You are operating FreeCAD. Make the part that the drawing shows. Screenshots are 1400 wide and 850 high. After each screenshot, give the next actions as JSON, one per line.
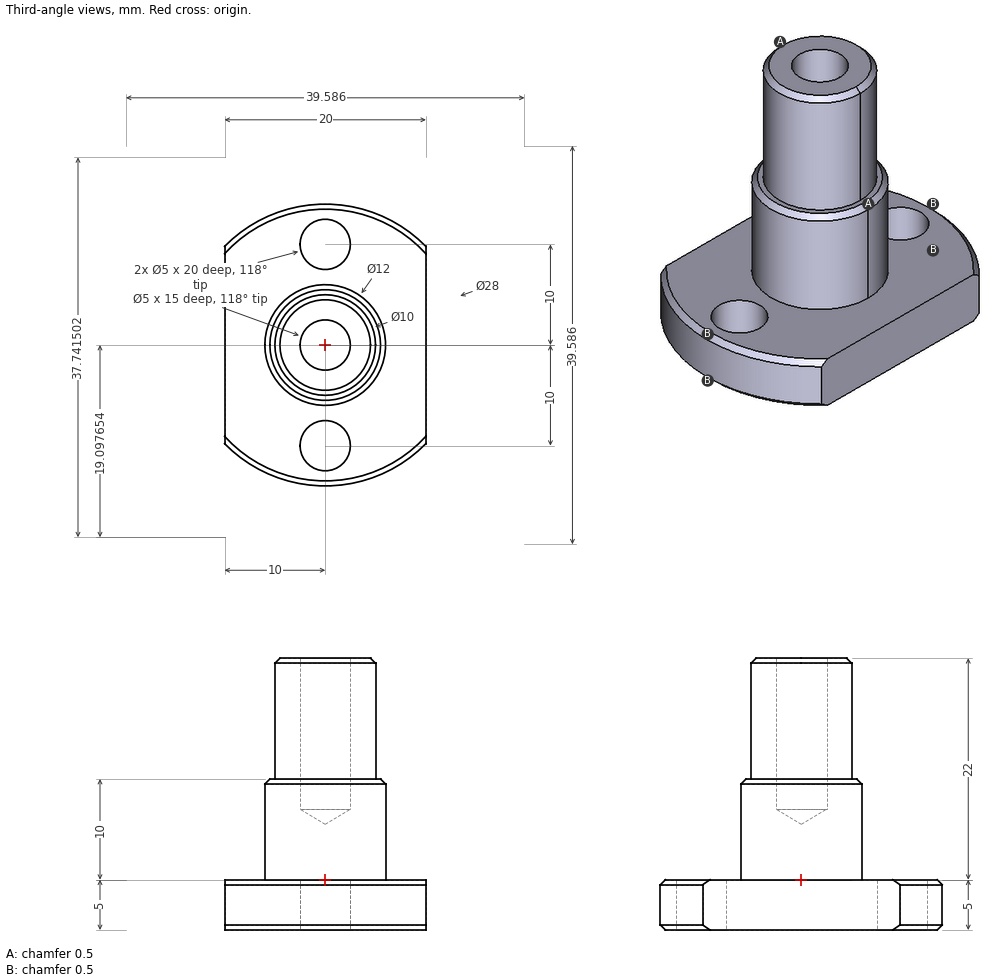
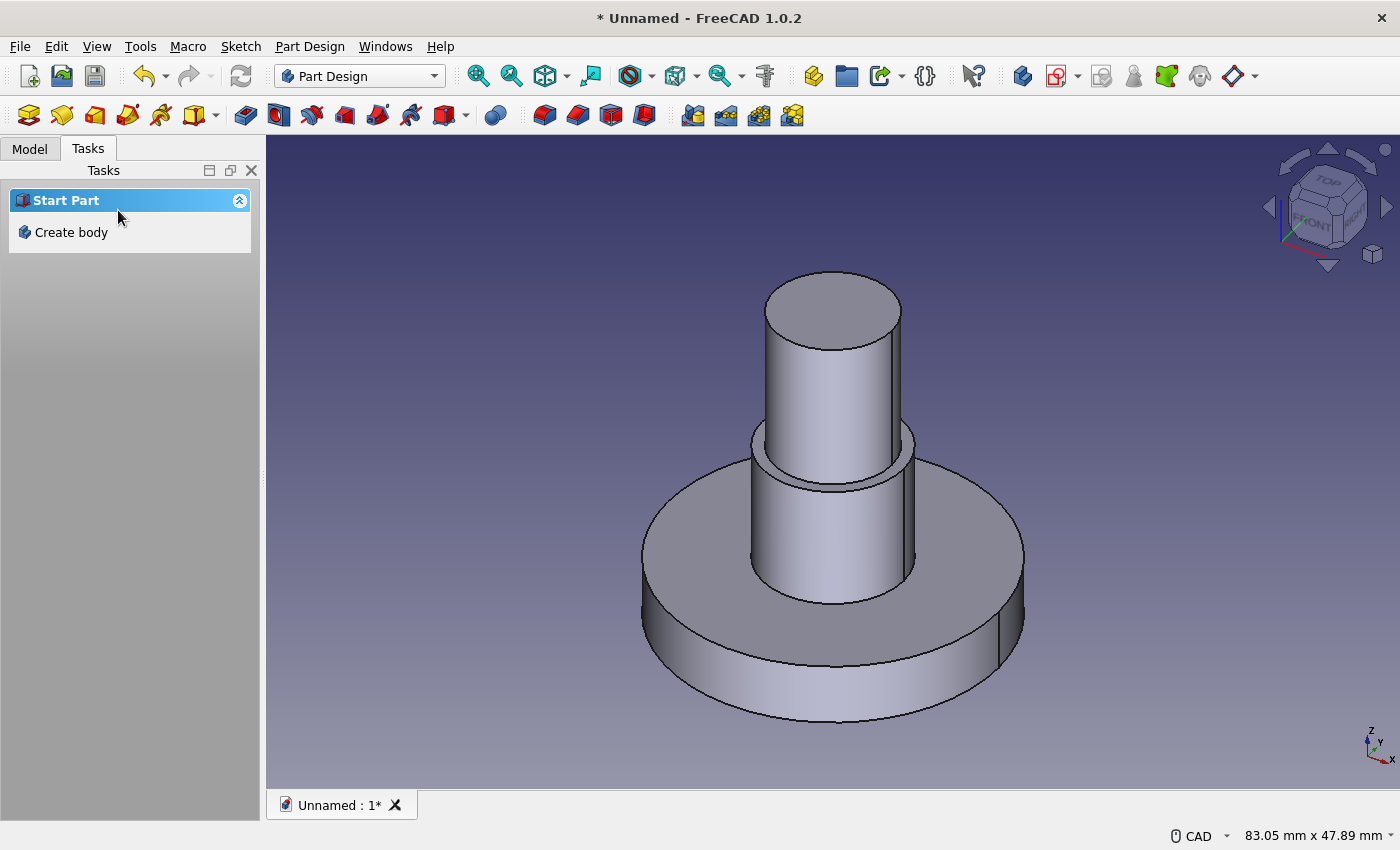
{"action": "key", "text": "5"}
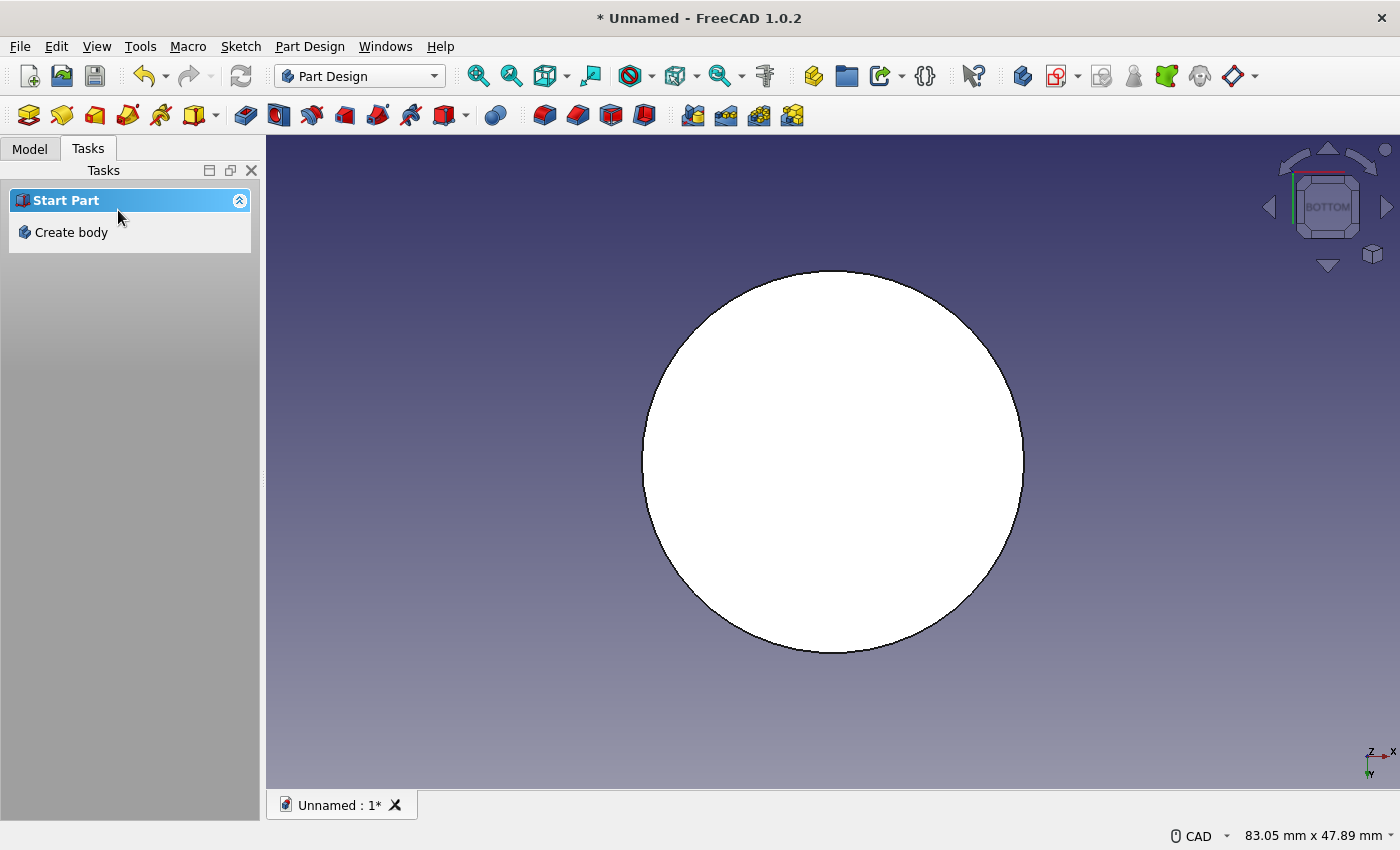
{"action": "left_click", "coordinate": [833, 461]}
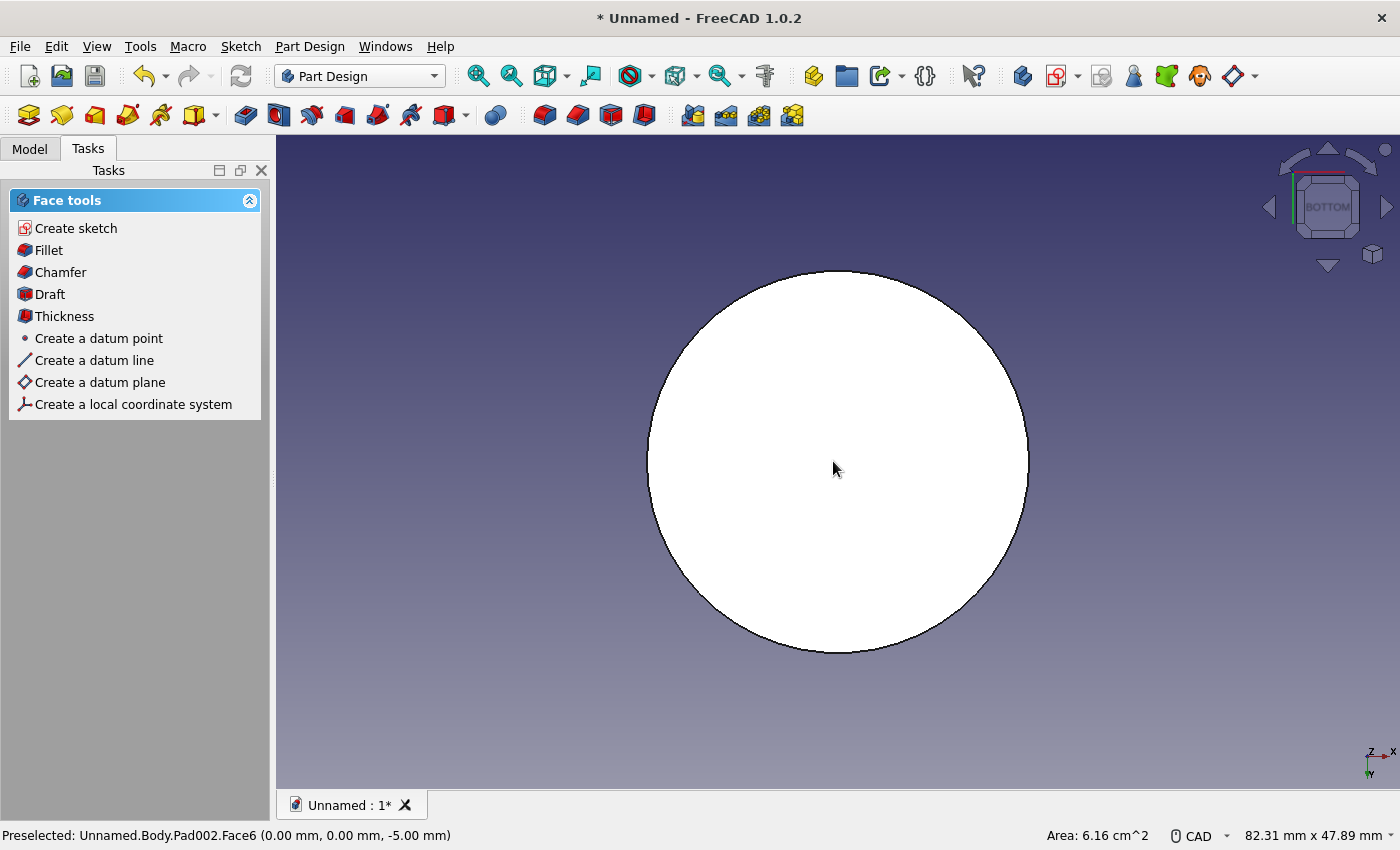
{"action": "left_click", "coordinate": [1056, 76]}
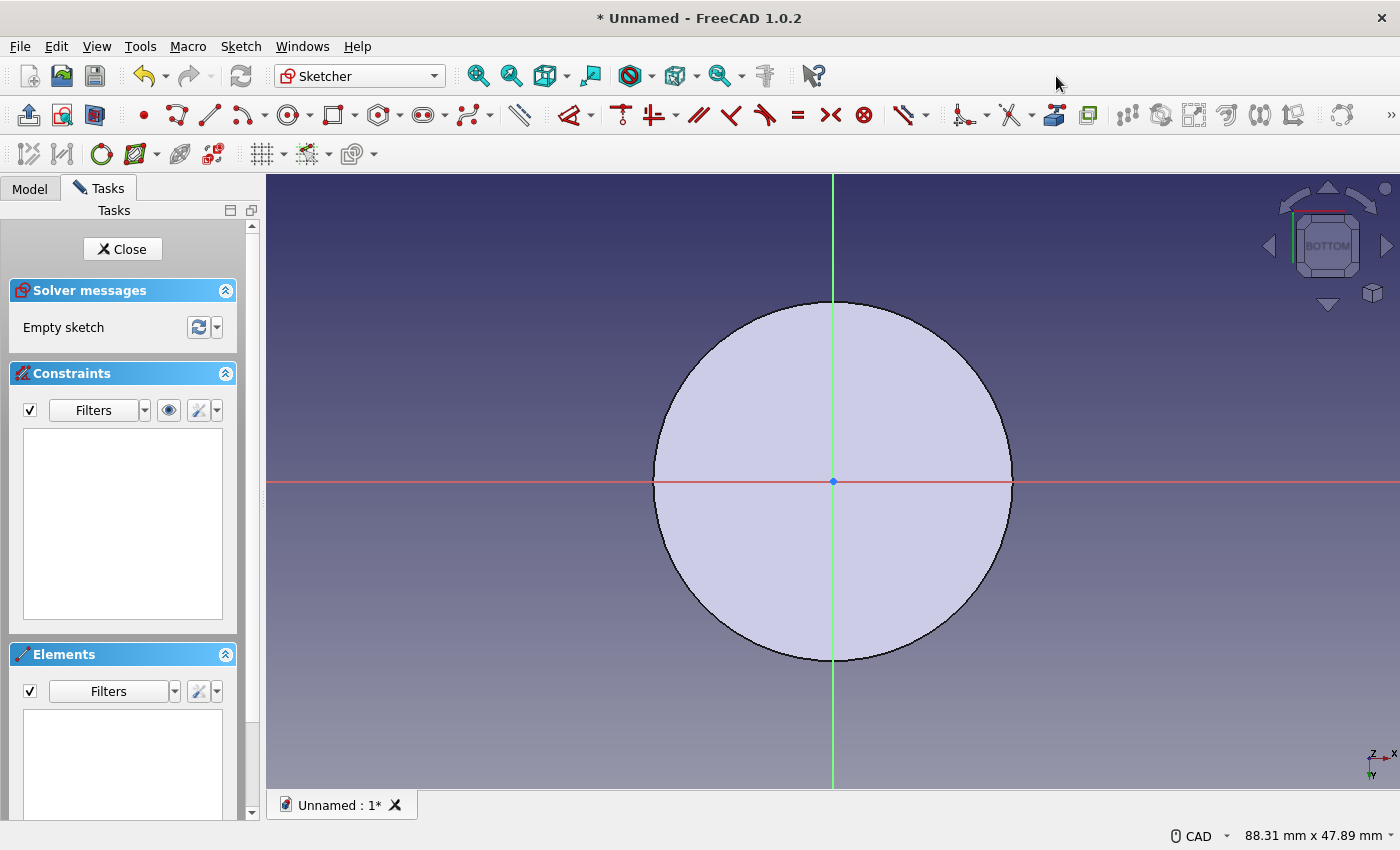
{"action": "key", "text": "g v"}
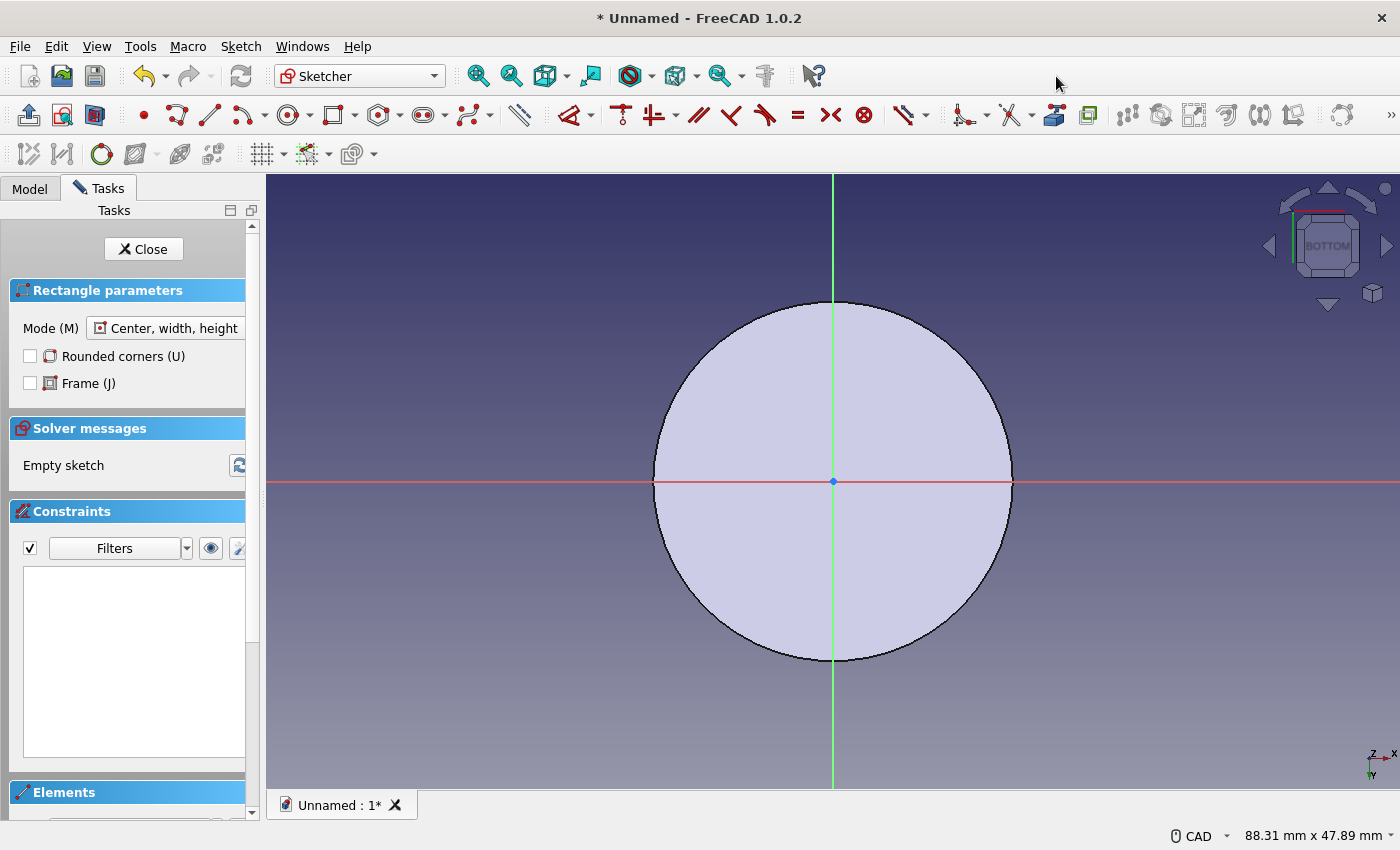
{"action": "left_click", "coordinate": [833, 482]}
{"action": "mouse_move", "coordinate": [1087, 227]}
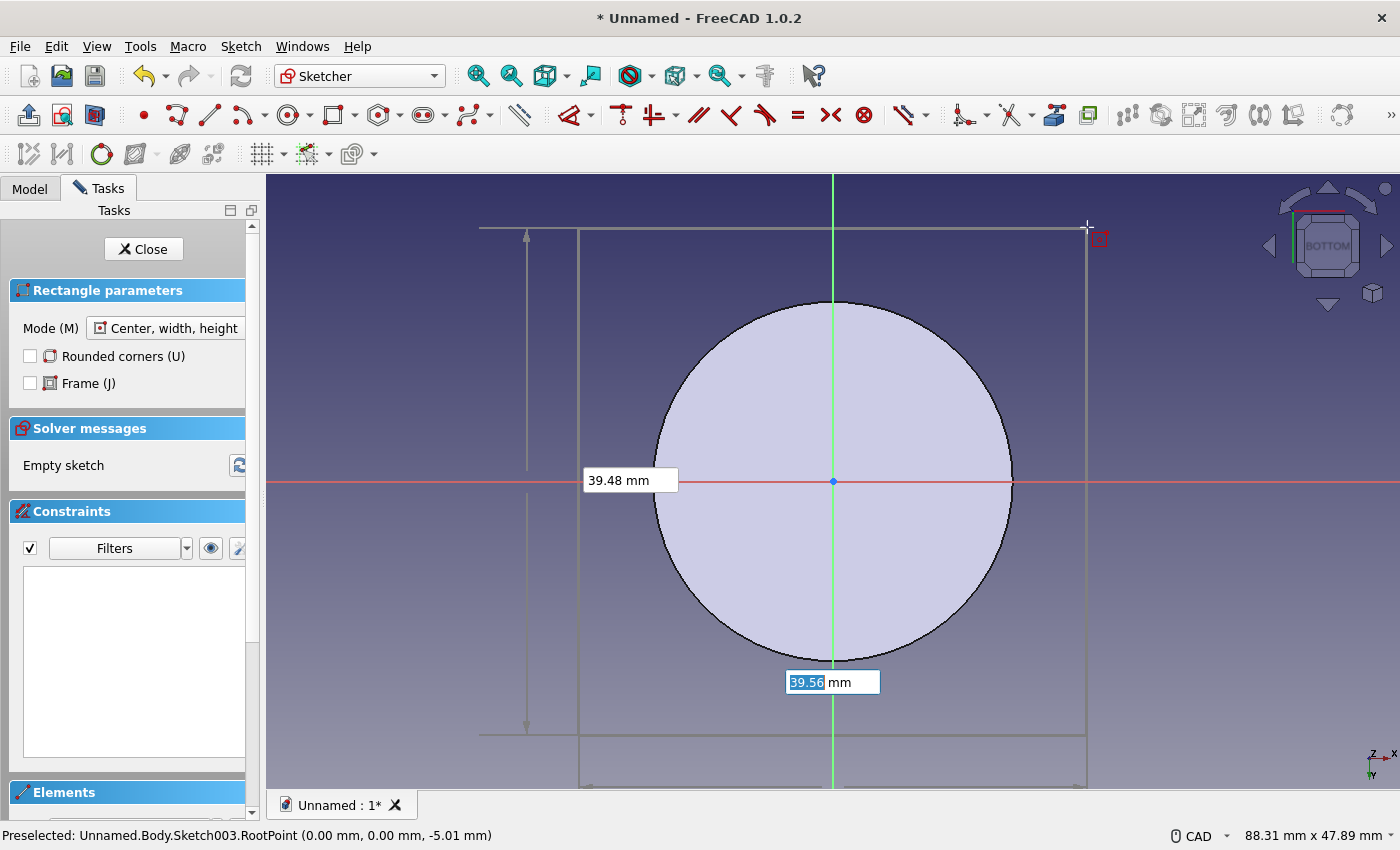
{"action": "type", "text": "39.586"}
{"action": "key", "text": "Tab"}
{"action": "type", "text": "39.586"}
{"action": "key", "text": "Return"}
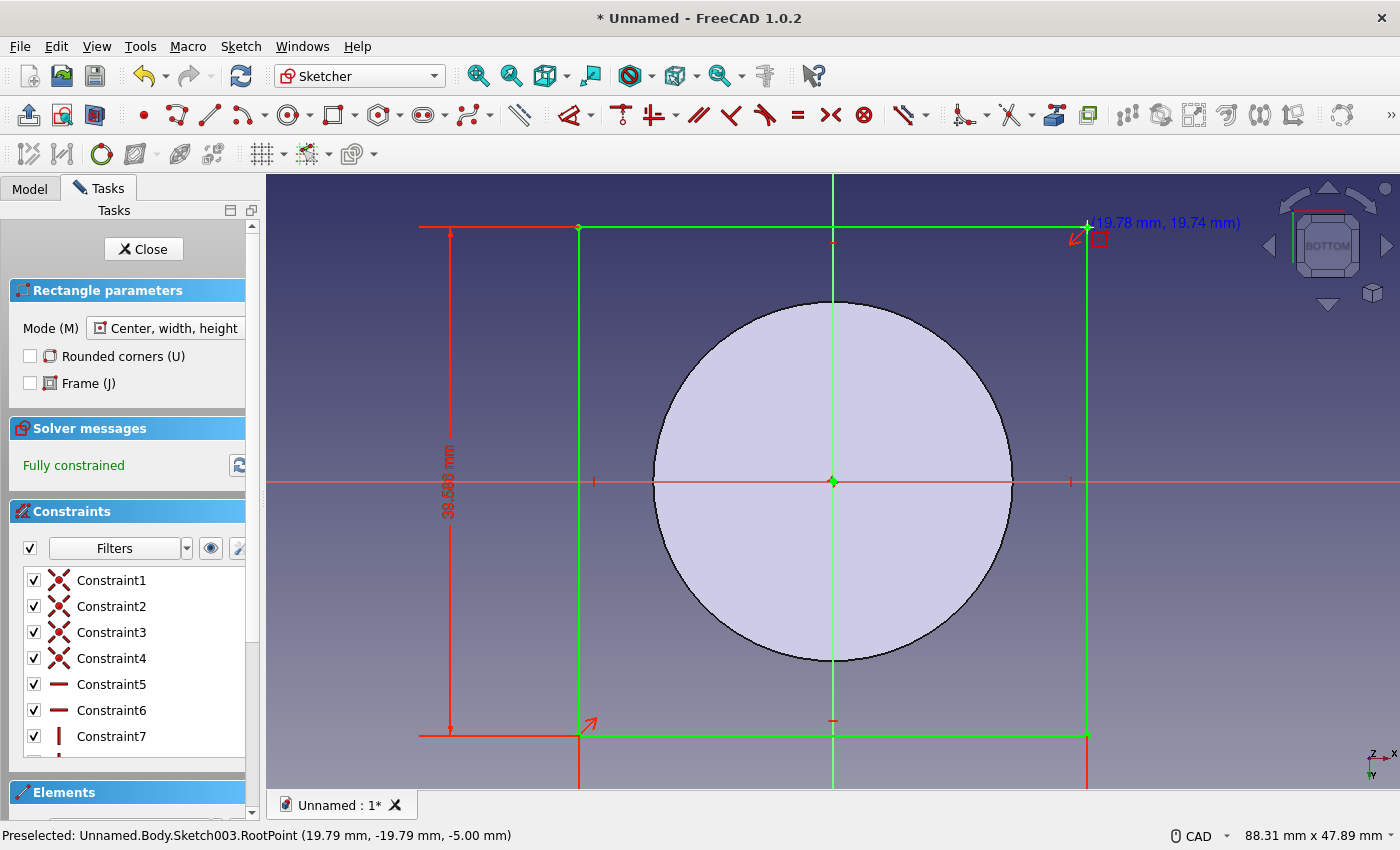
{"action": "key", "text": "g r"}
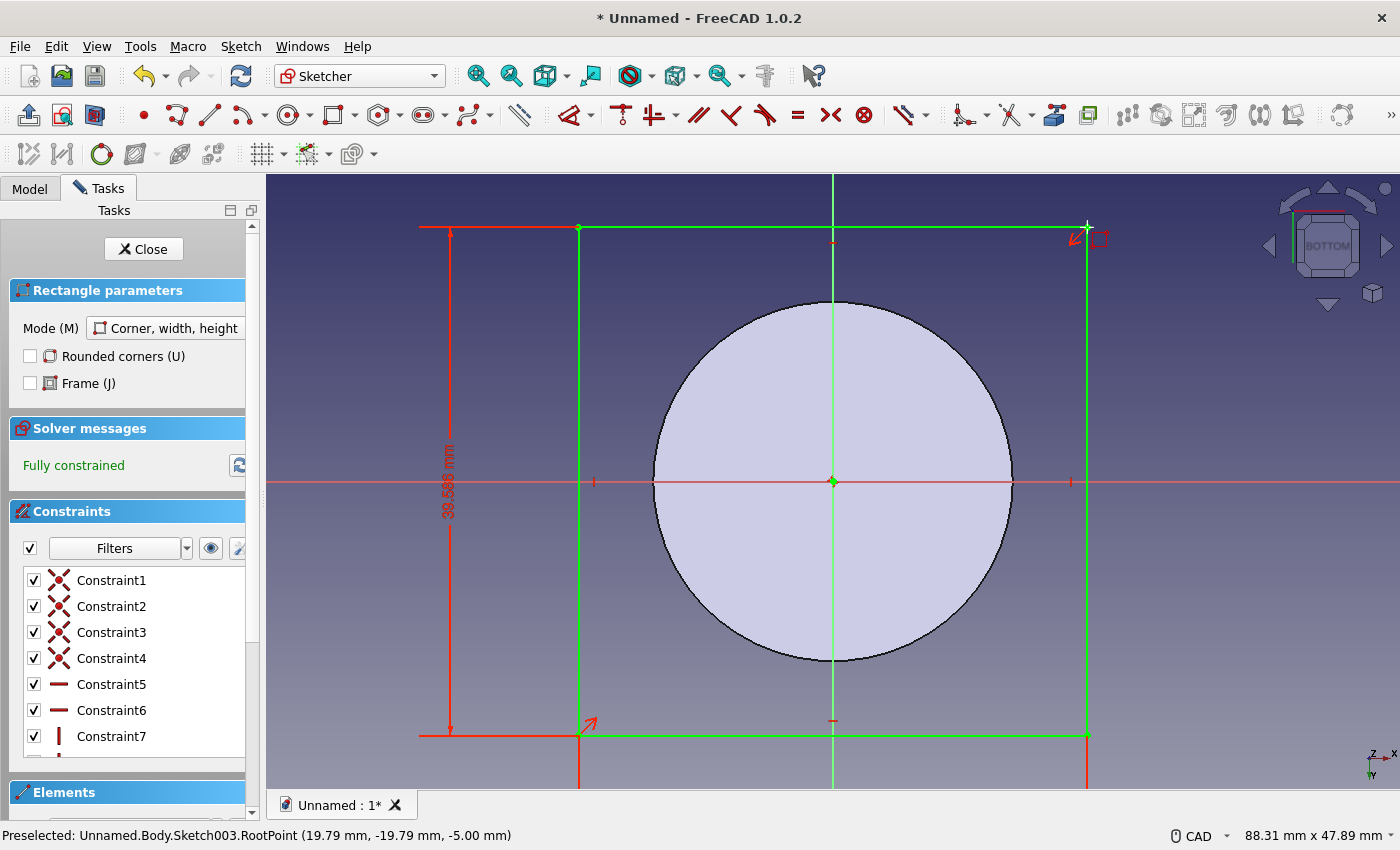
{"action": "scroll", "coordinate": [705, 236], "scroll_direction": "up", "scroll_amount": 3}